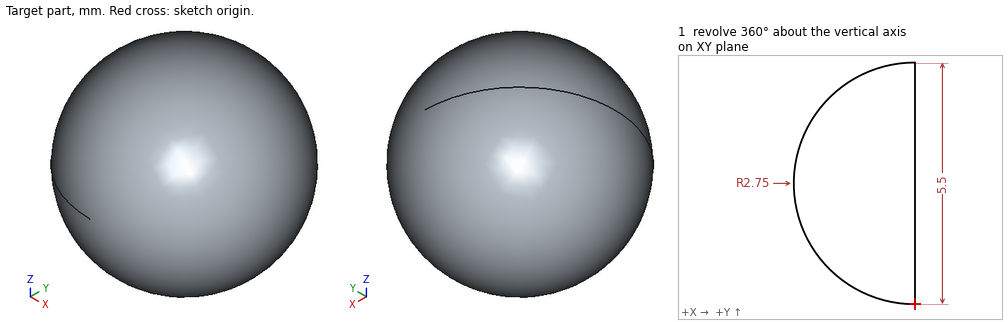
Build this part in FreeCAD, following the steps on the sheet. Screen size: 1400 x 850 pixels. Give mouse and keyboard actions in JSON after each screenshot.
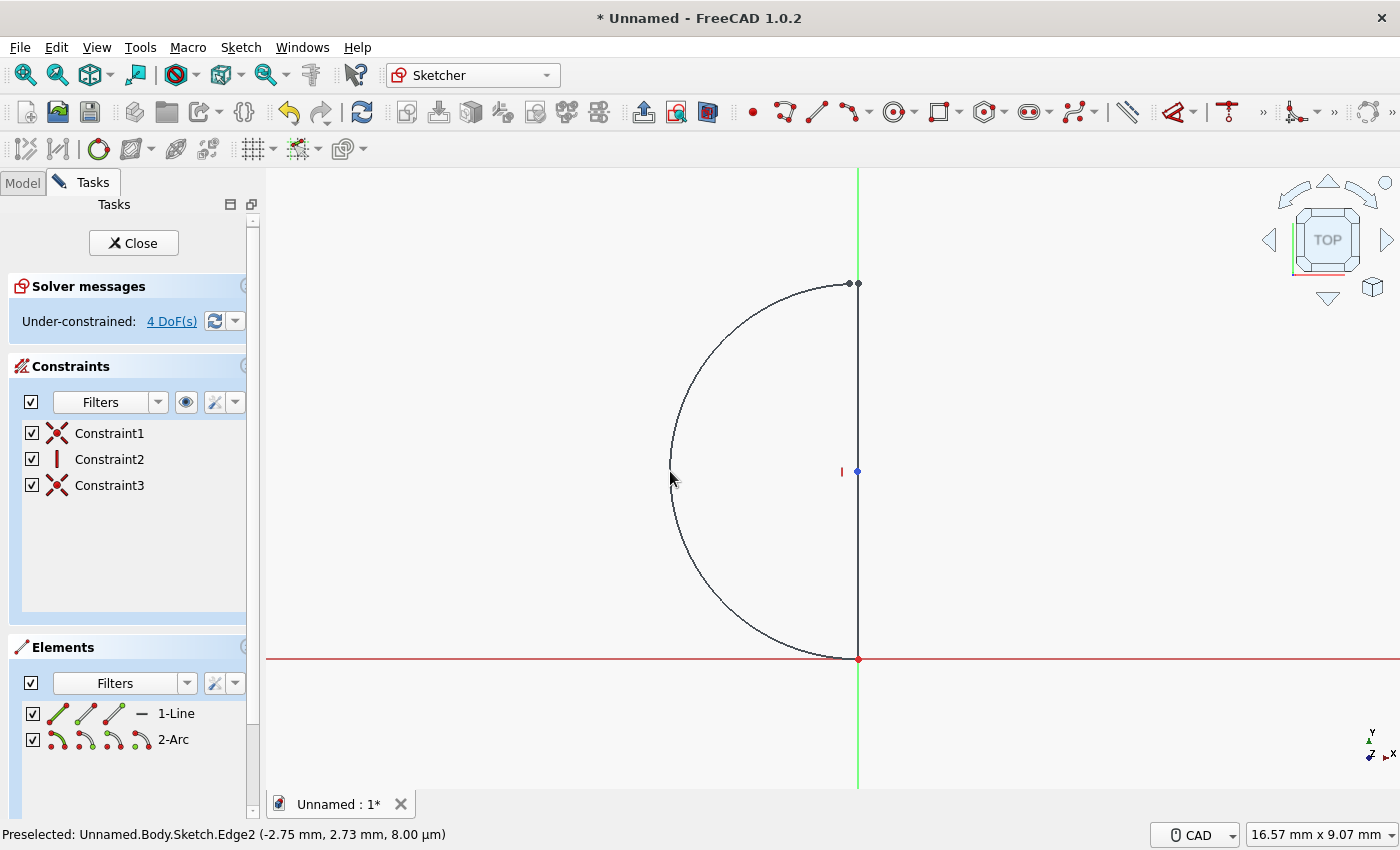
{"action": "left_click", "coordinate": [858, 472]}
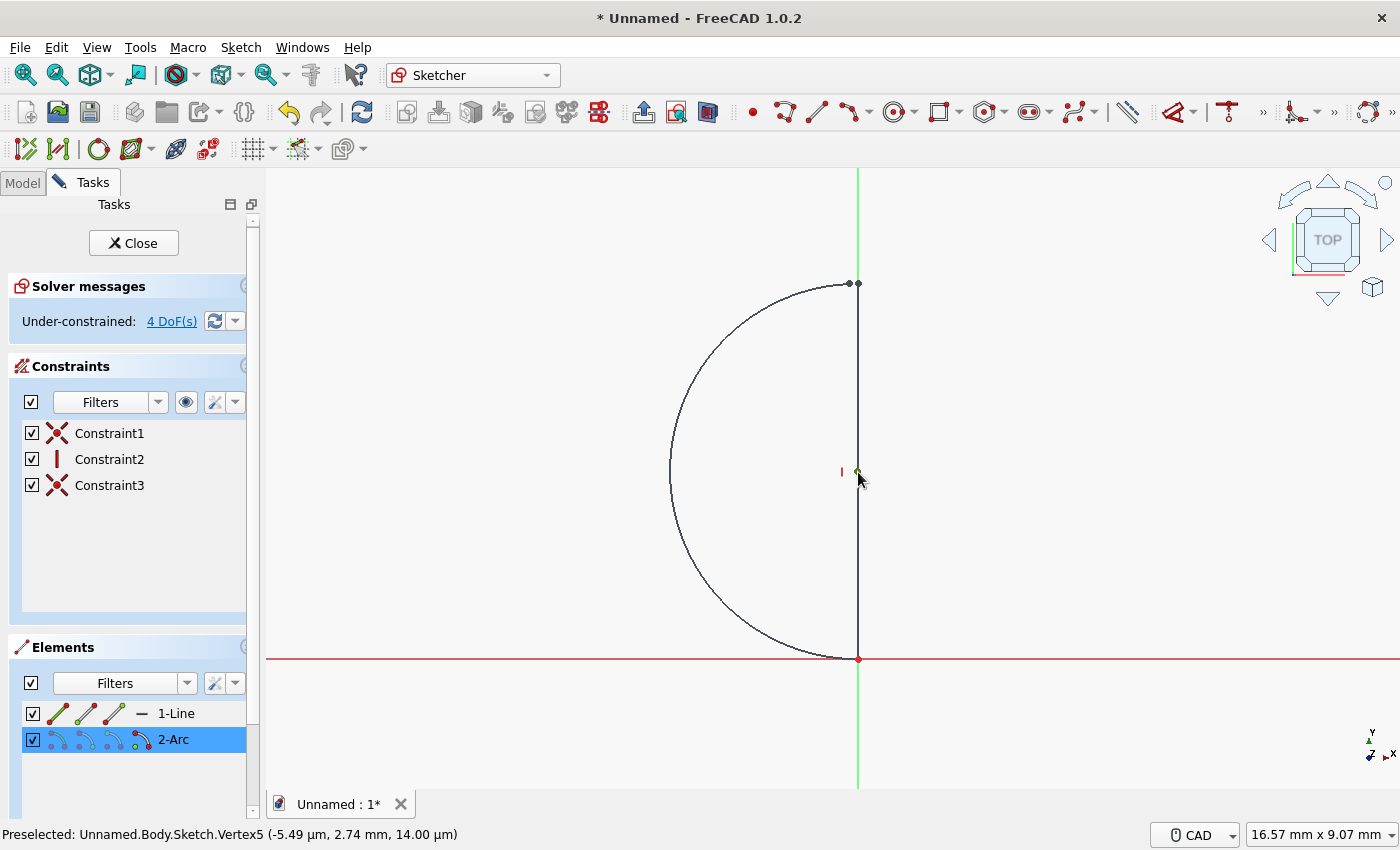
{"action": "left_click", "coordinate": [858, 721]}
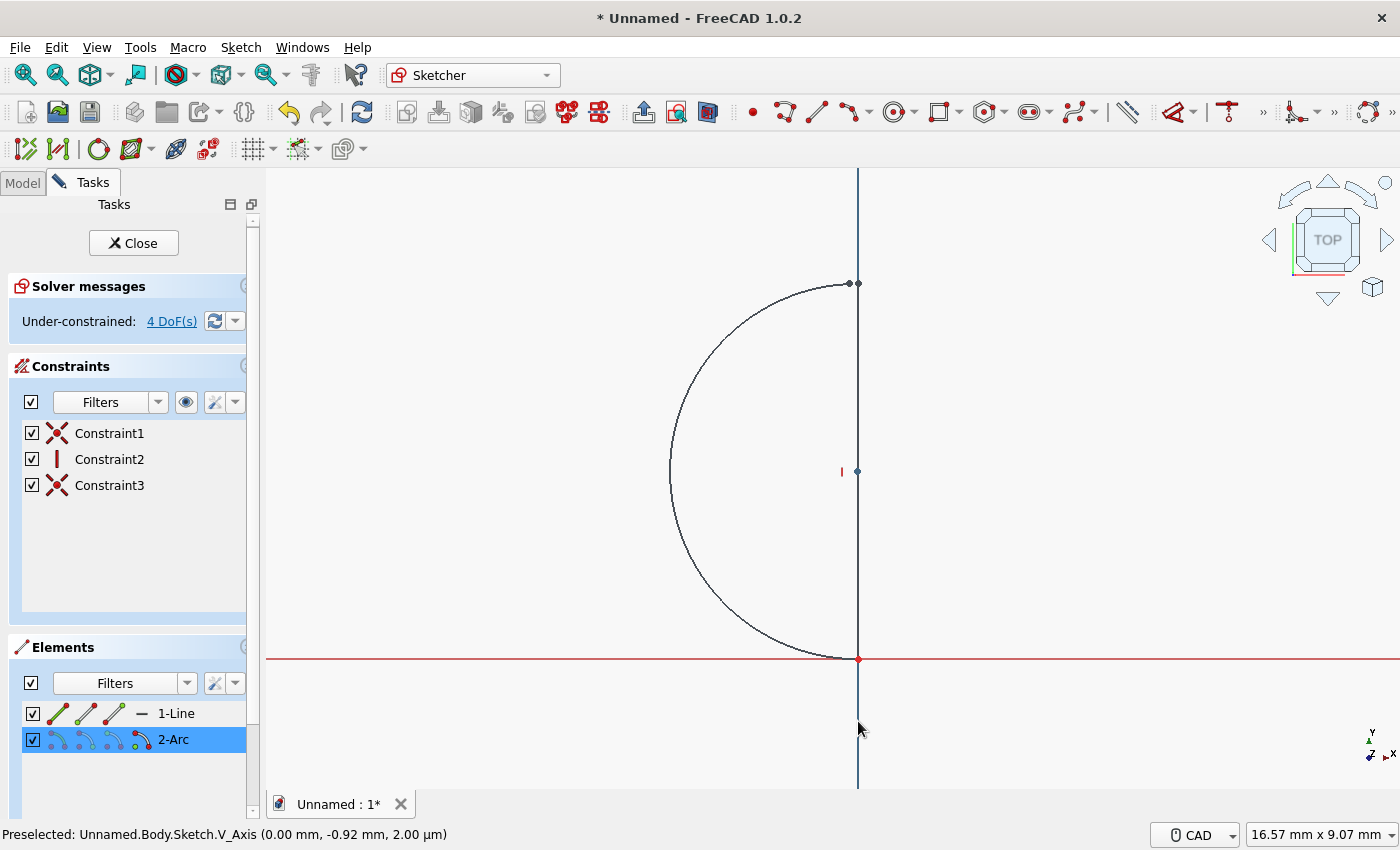
{"action": "left_click", "coordinate": [1228, 112]}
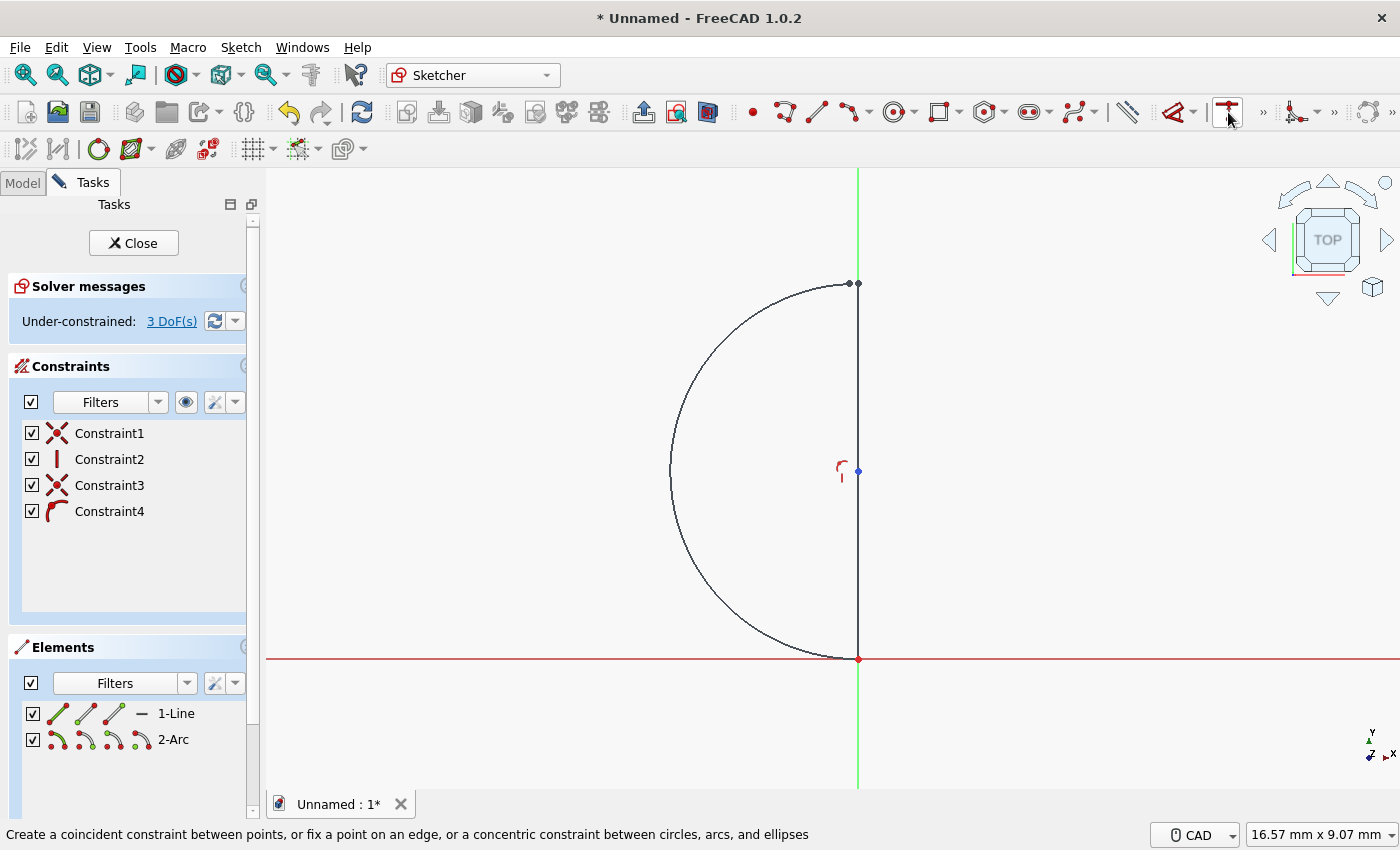
{"action": "left_click", "coordinate": [1174, 112]}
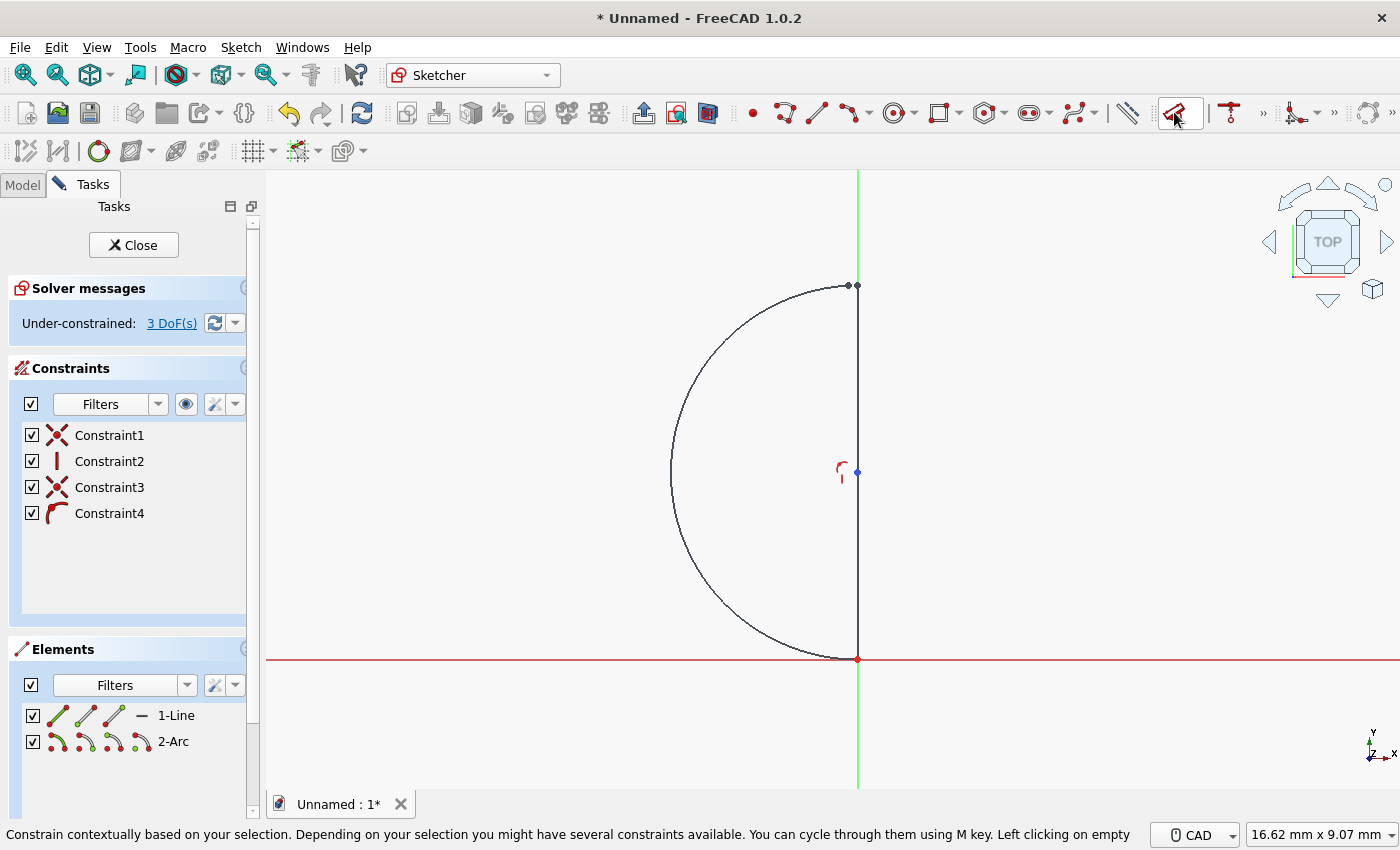
{"action": "left_click", "coordinate": [703, 368]}
{"action": "left_click", "coordinate": [676, 350]}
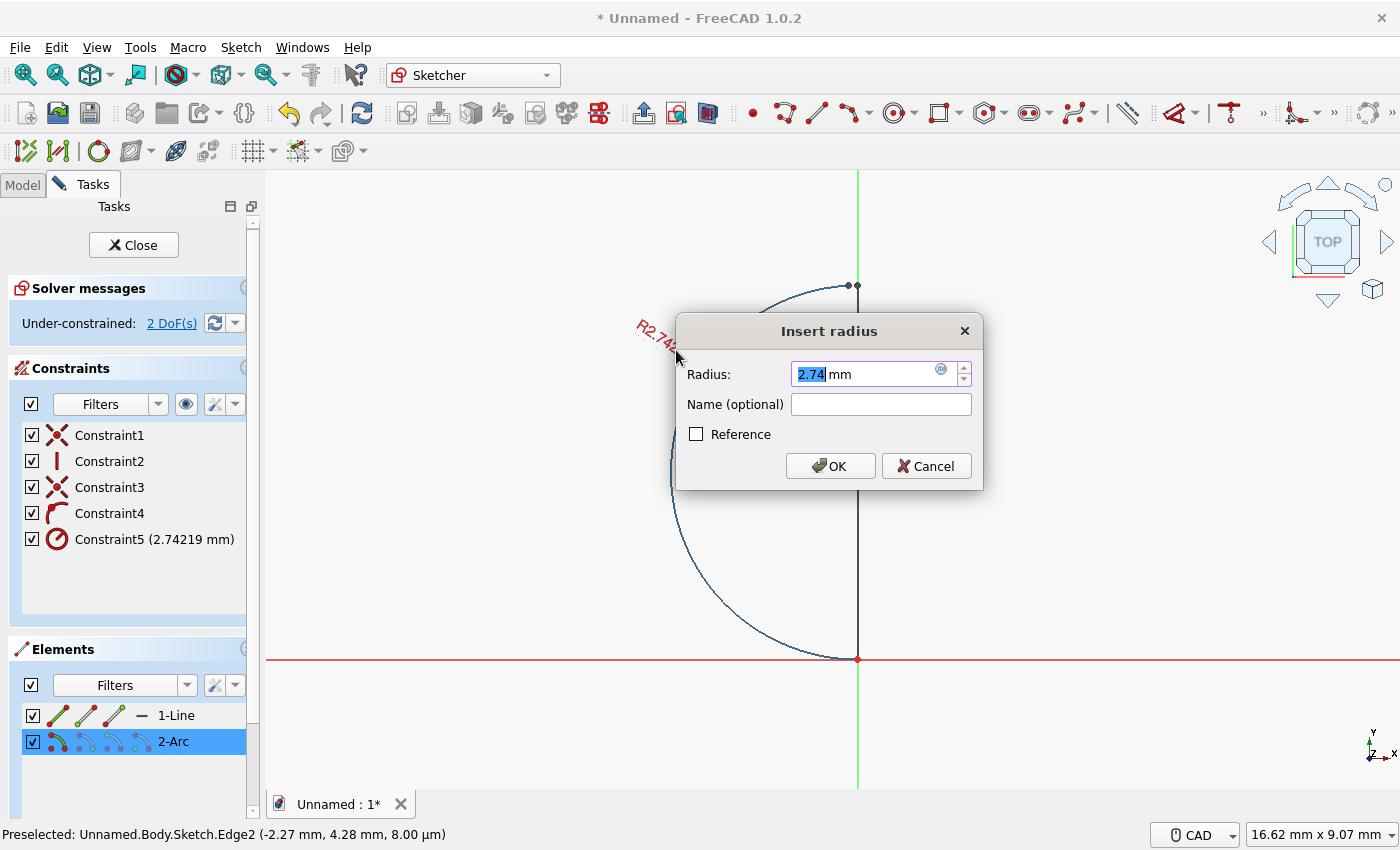
{"action": "type", "text": "2.75"}
{"action": "key", "text": "Return"}
{"action": "key", "text": "Escape"}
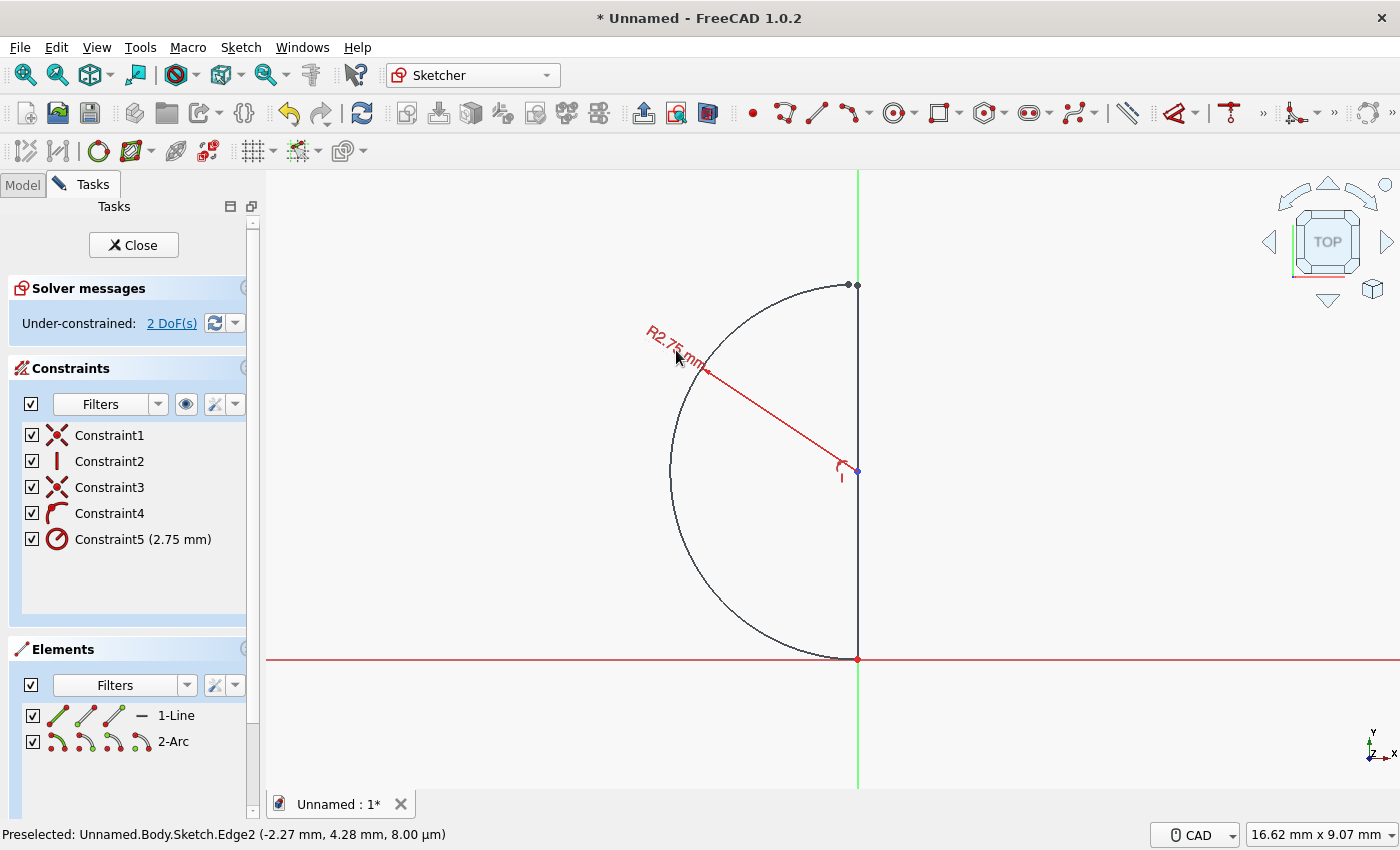
{"action": "left_click", "coordinate": [849, 285]}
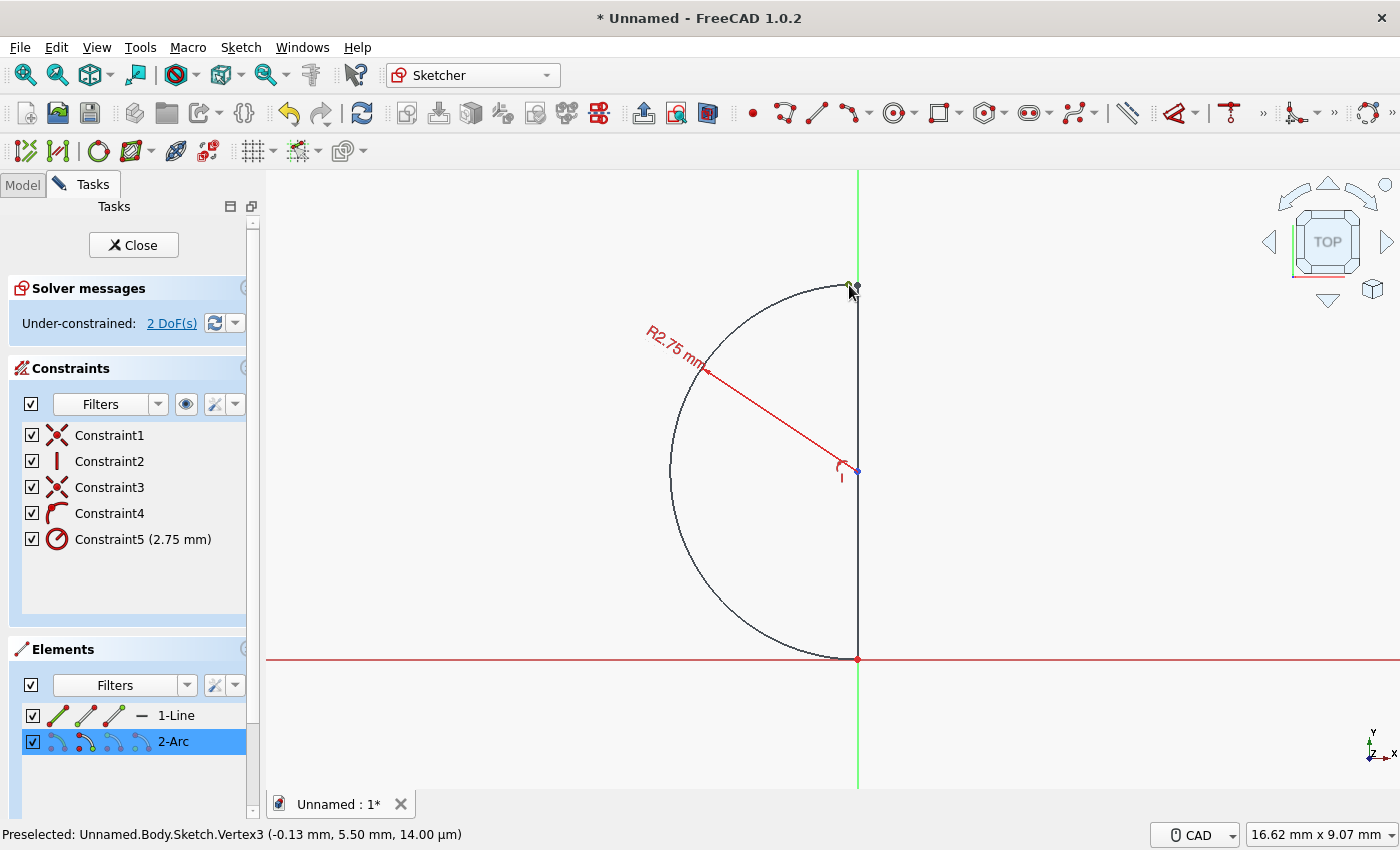
{"action": "left_click", "coordinate": [858, 721]}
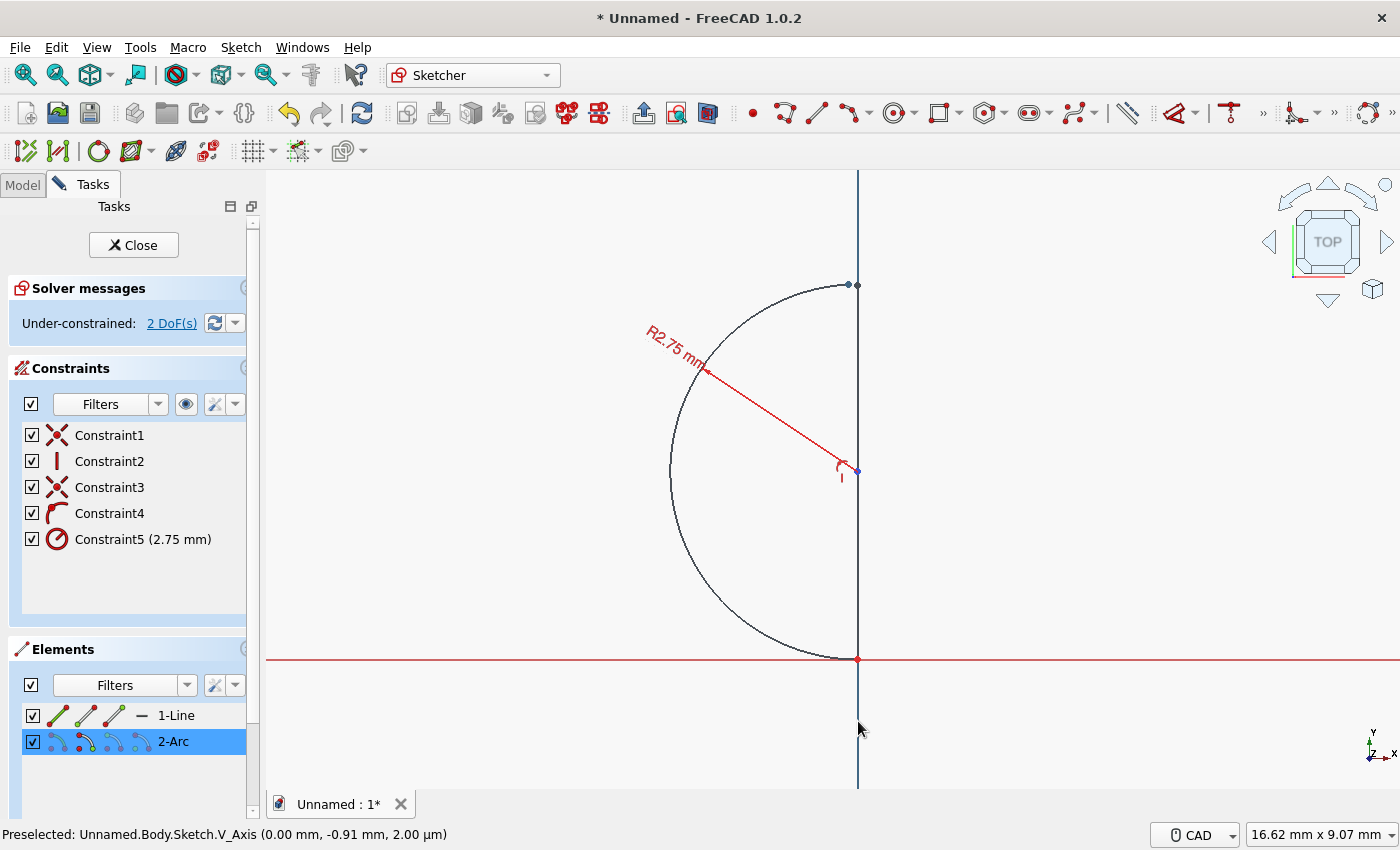
{"action": "left_click", "coordinate": [1230, 114]}